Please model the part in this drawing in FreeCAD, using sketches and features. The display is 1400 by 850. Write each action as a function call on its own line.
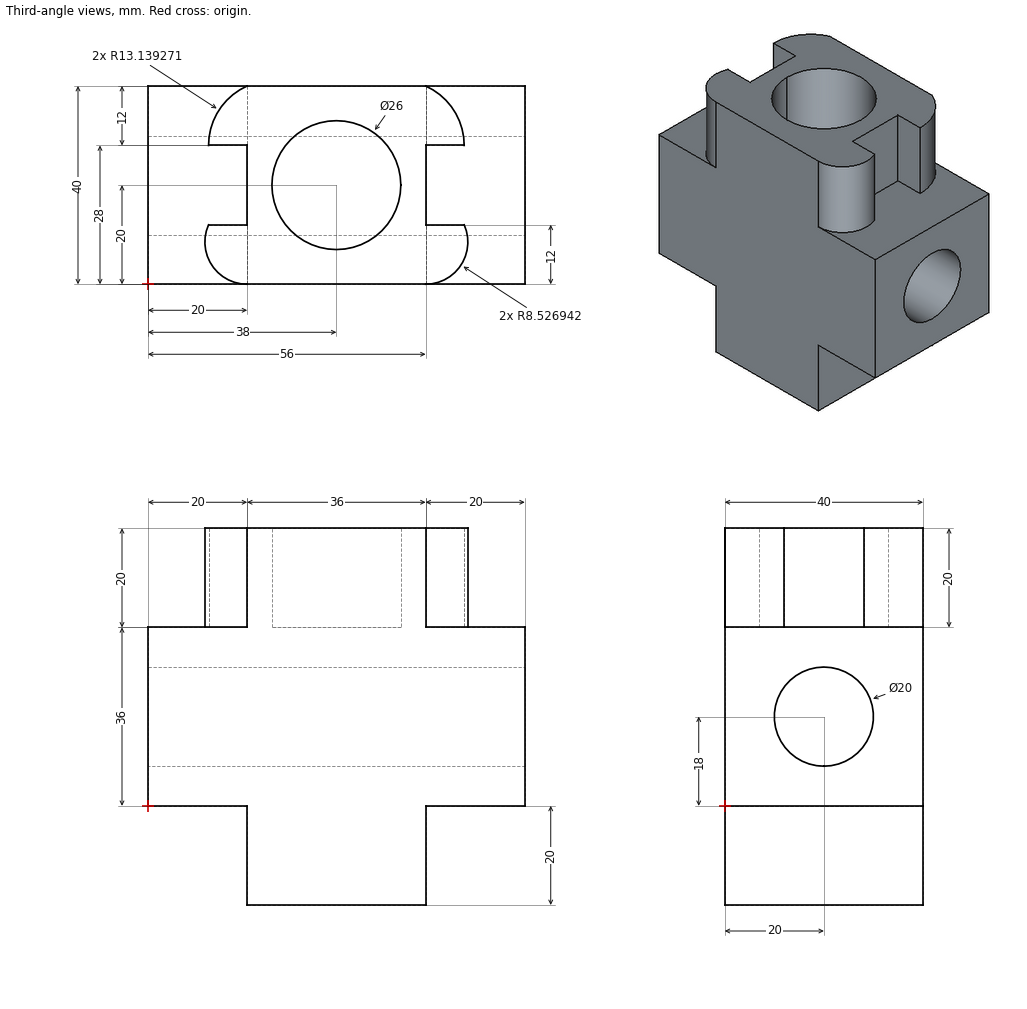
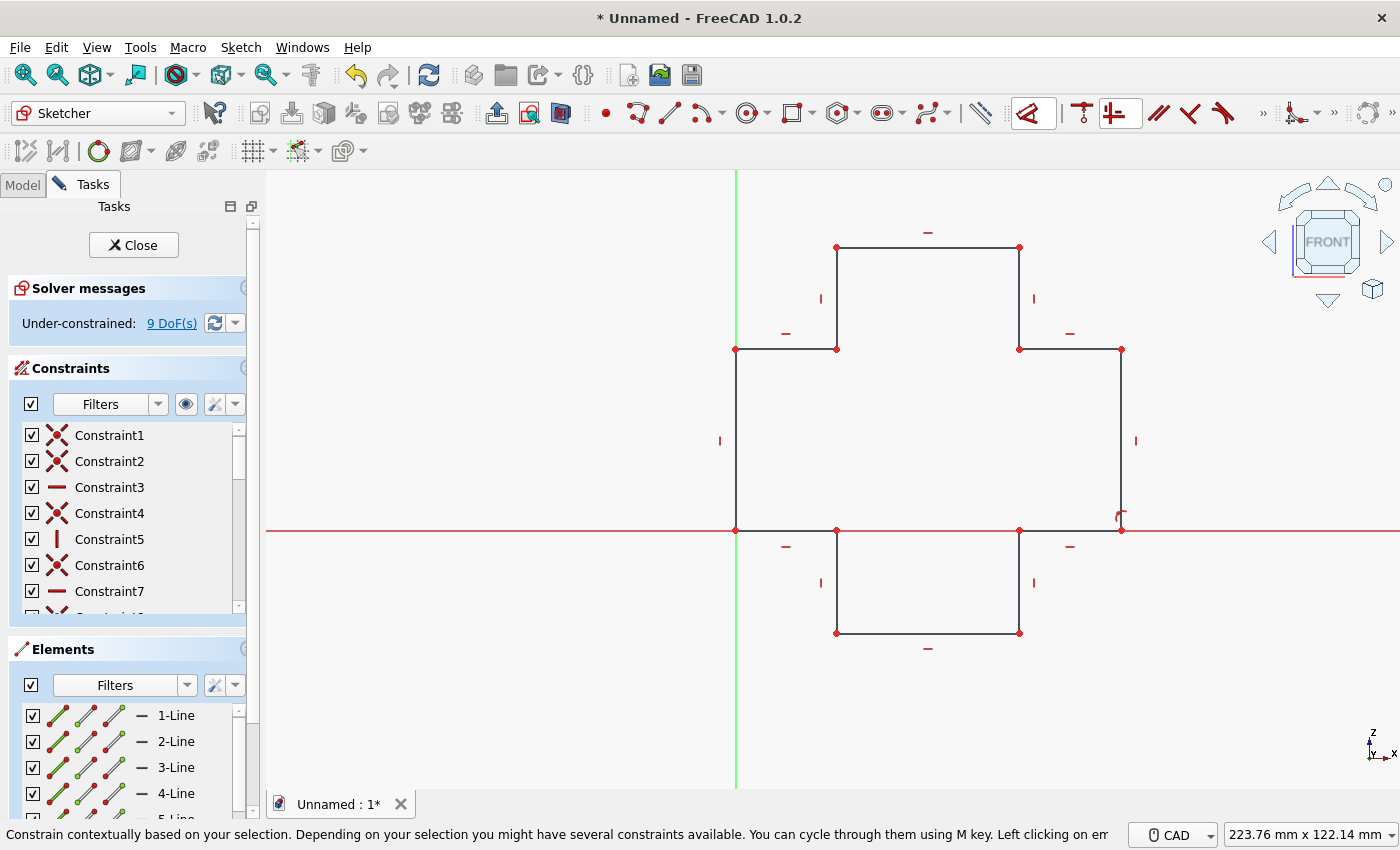
click(736, 476)
click(702, 440)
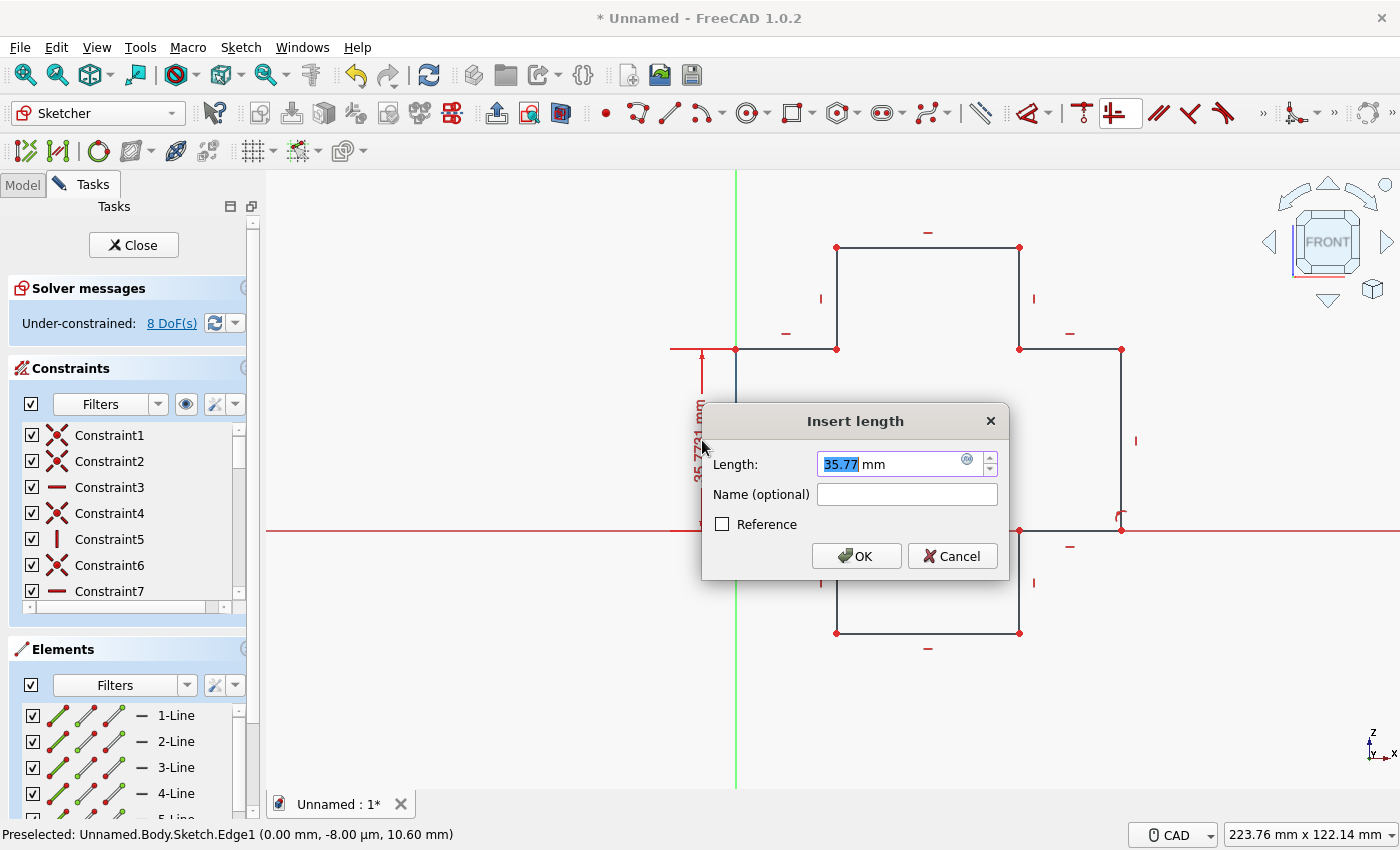
text(36)
key(Return)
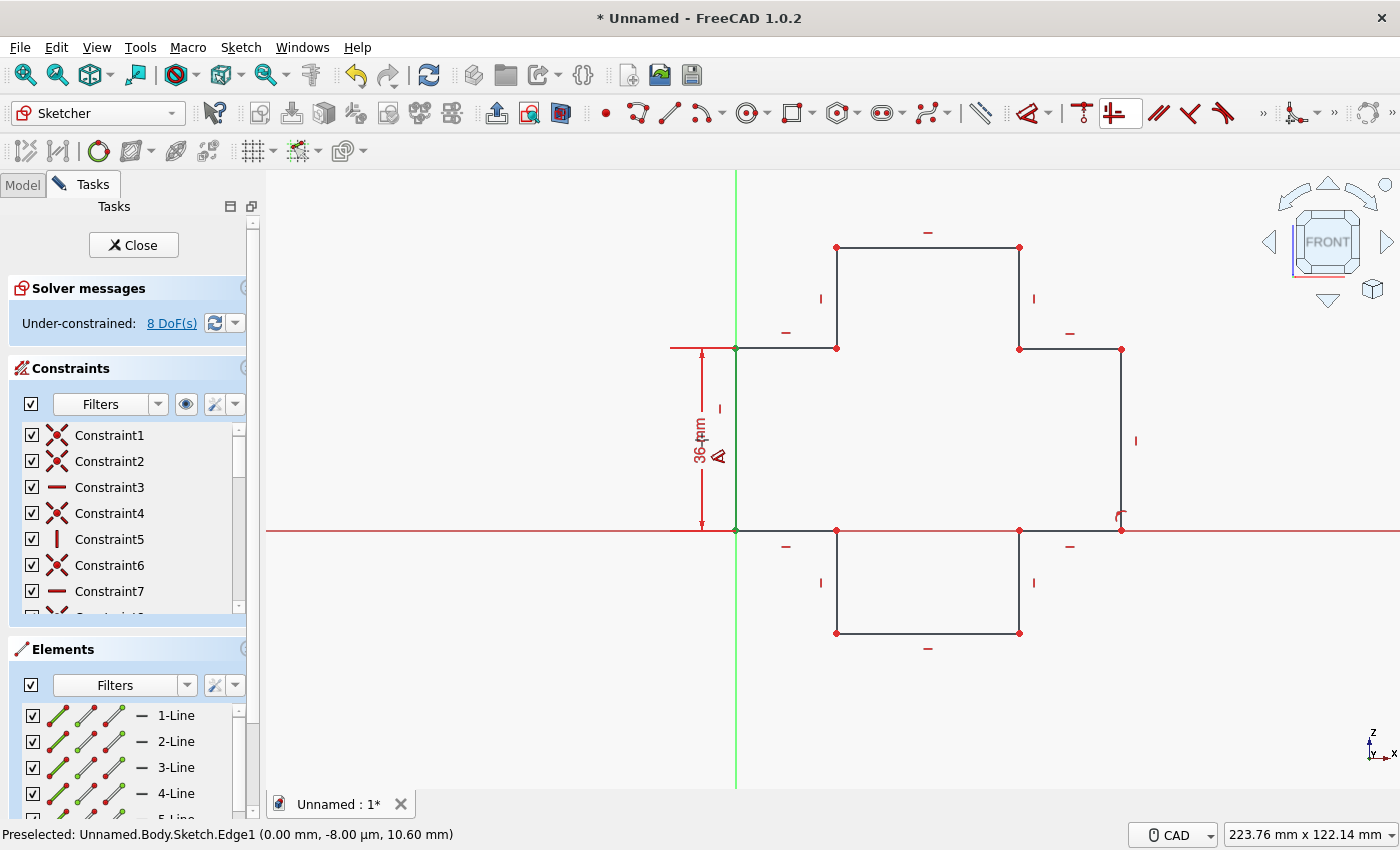
click(766, 348)
click(786, 314)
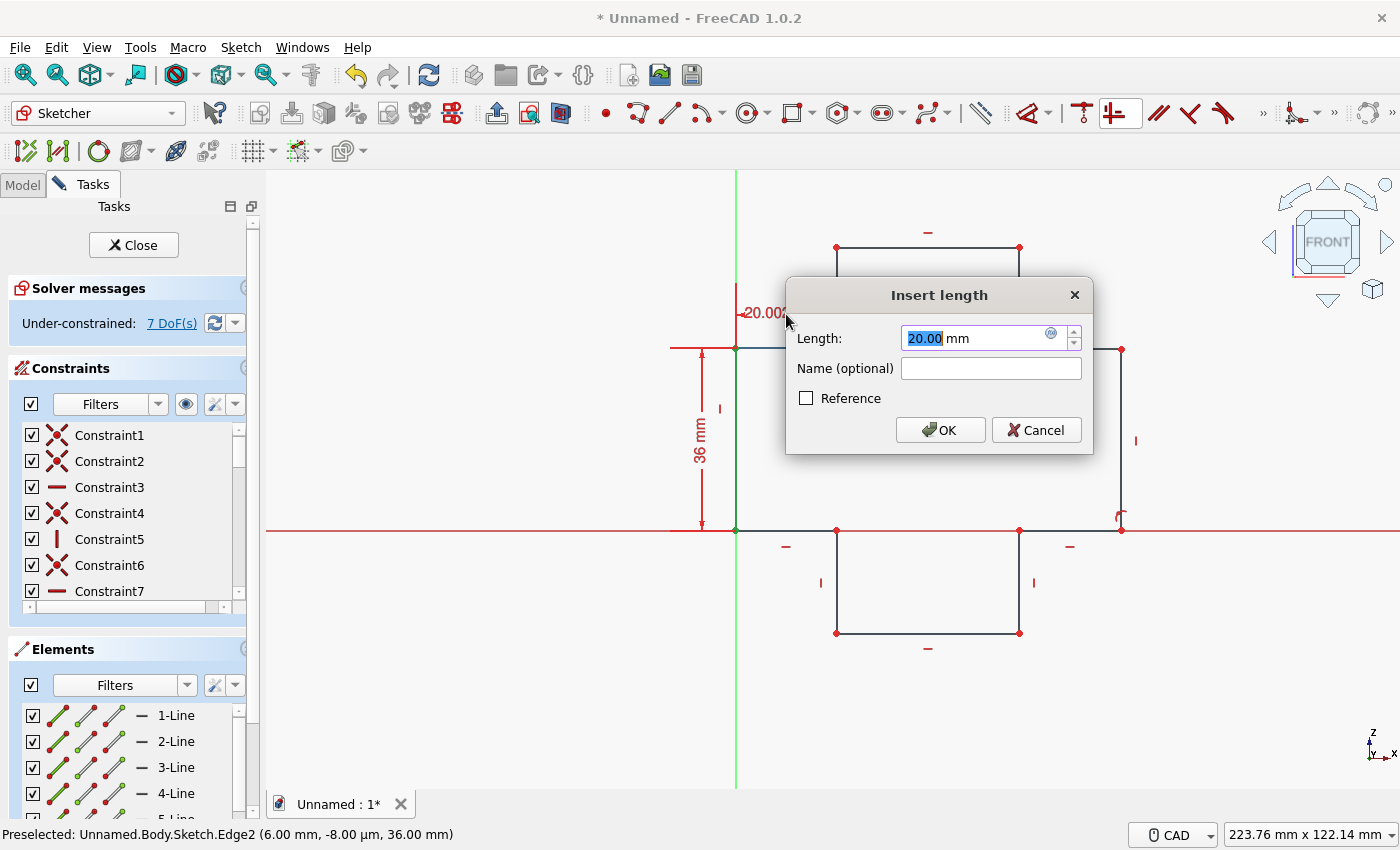
text(20)
key(Return)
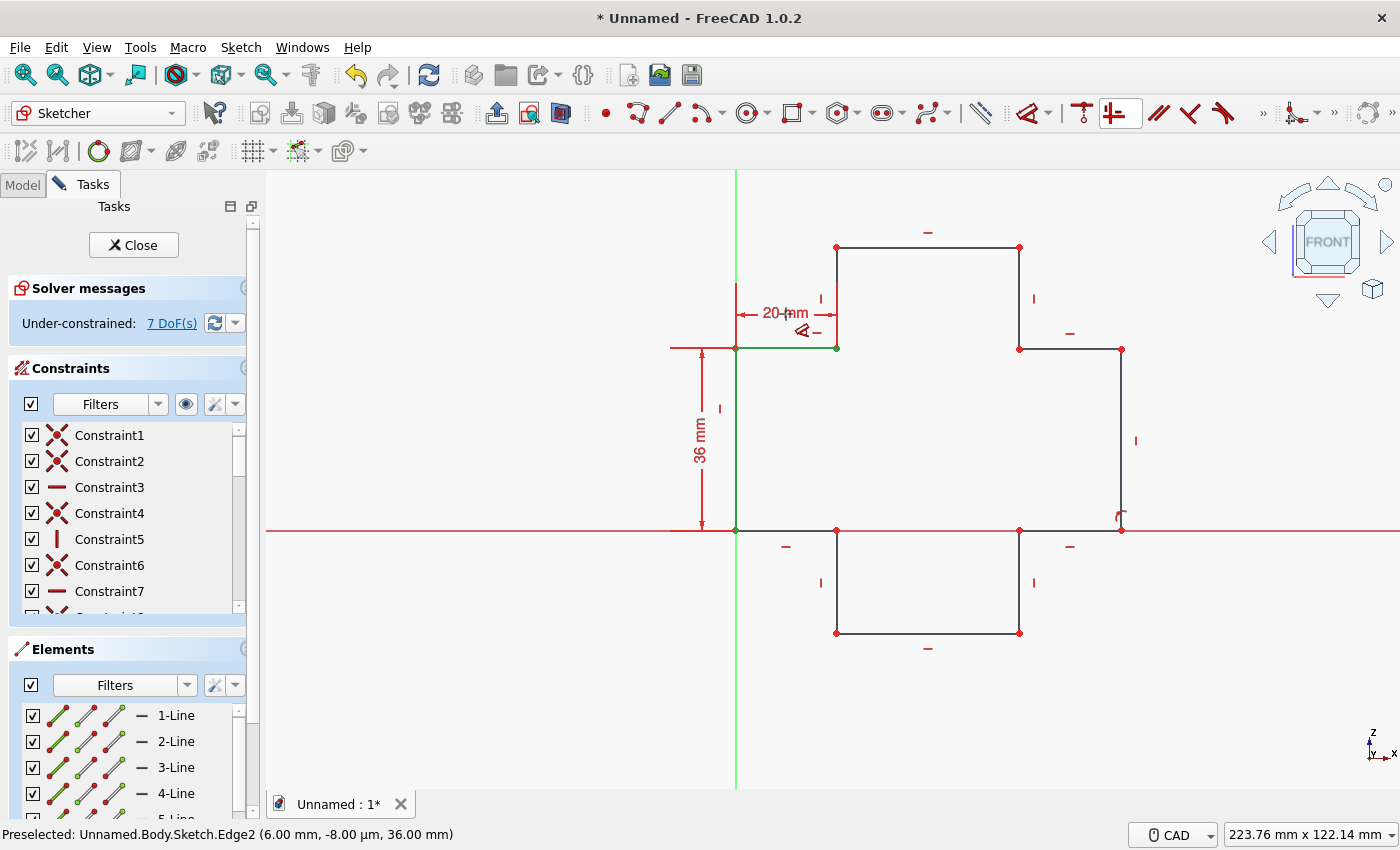
click(837, 318)
click(803, 275)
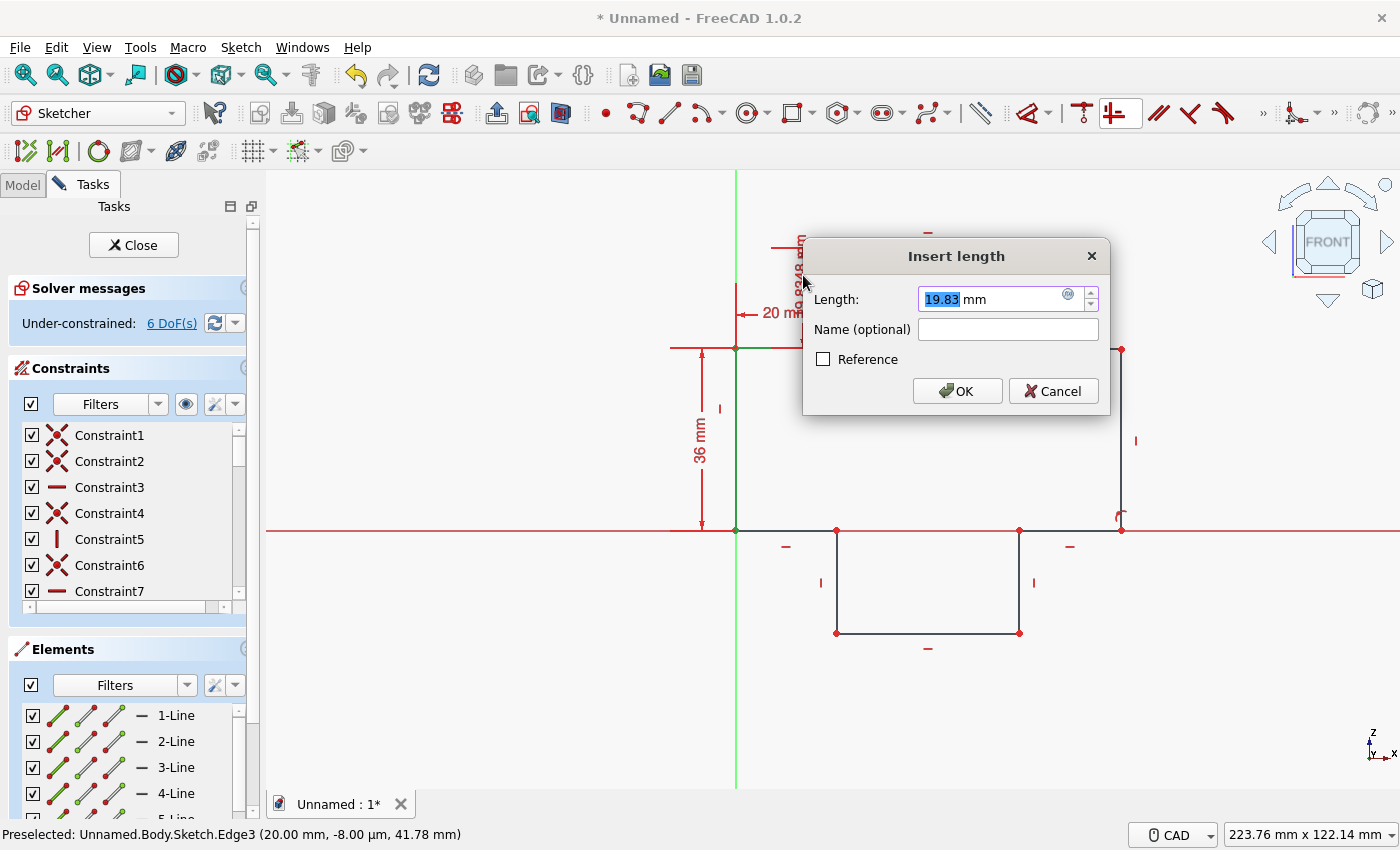
text(20)
key(Return)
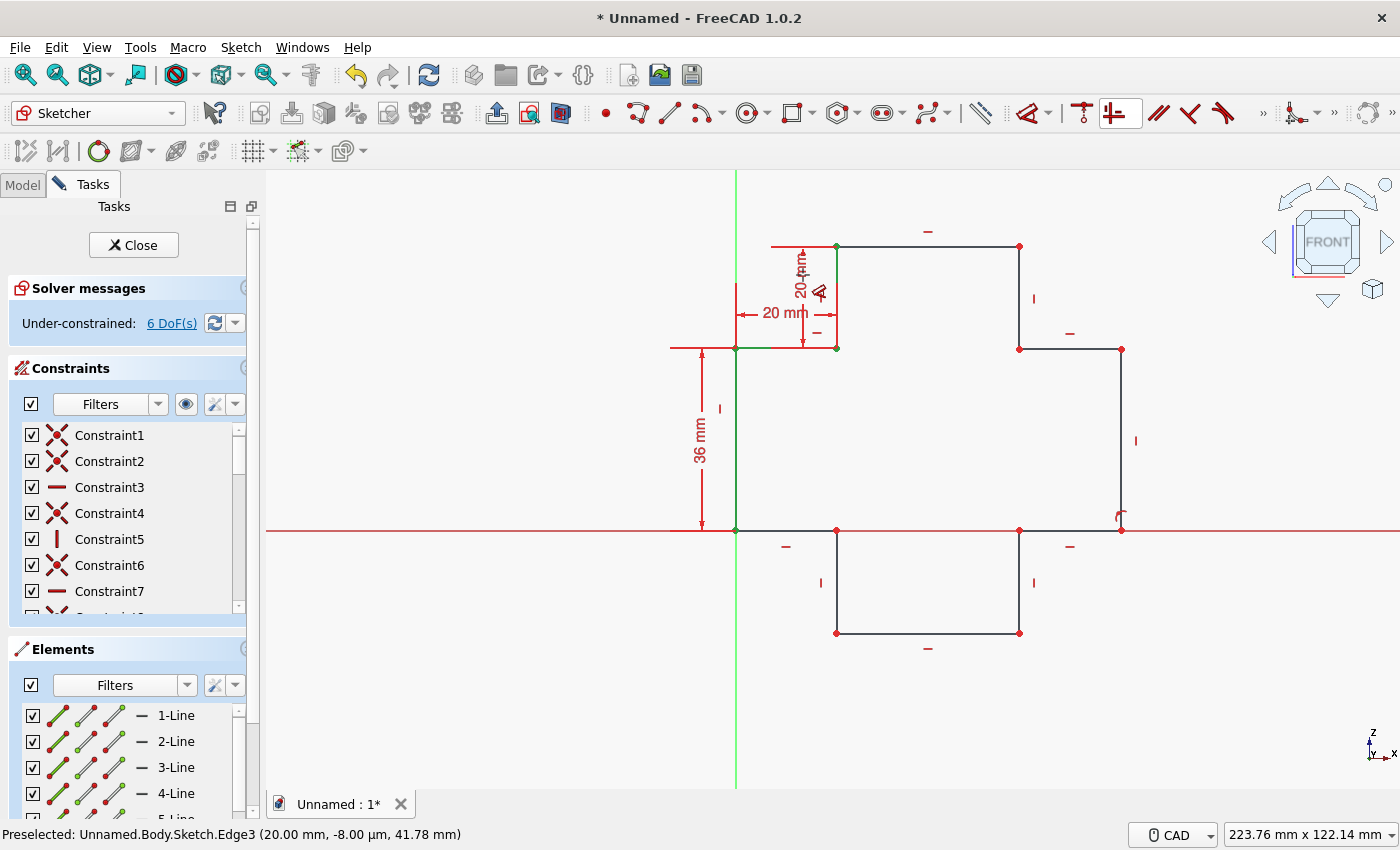
click(892, 247)
click(928, 213)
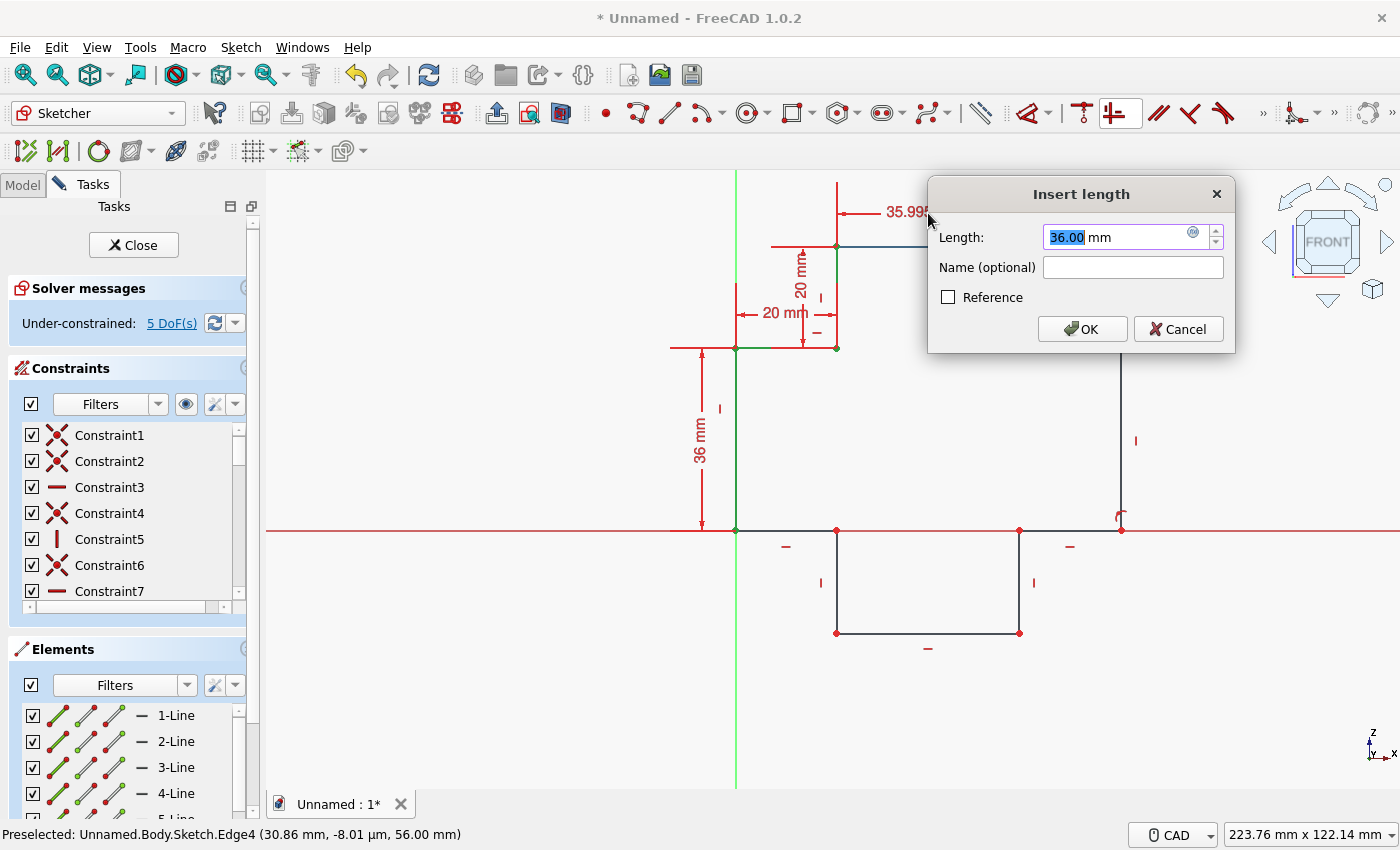
text(36)
key(Return)